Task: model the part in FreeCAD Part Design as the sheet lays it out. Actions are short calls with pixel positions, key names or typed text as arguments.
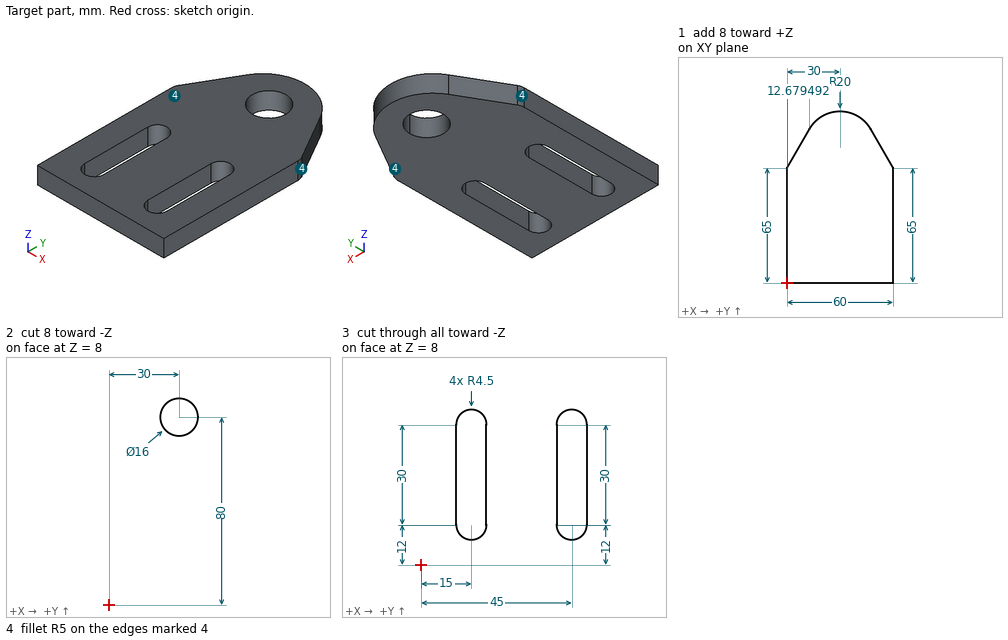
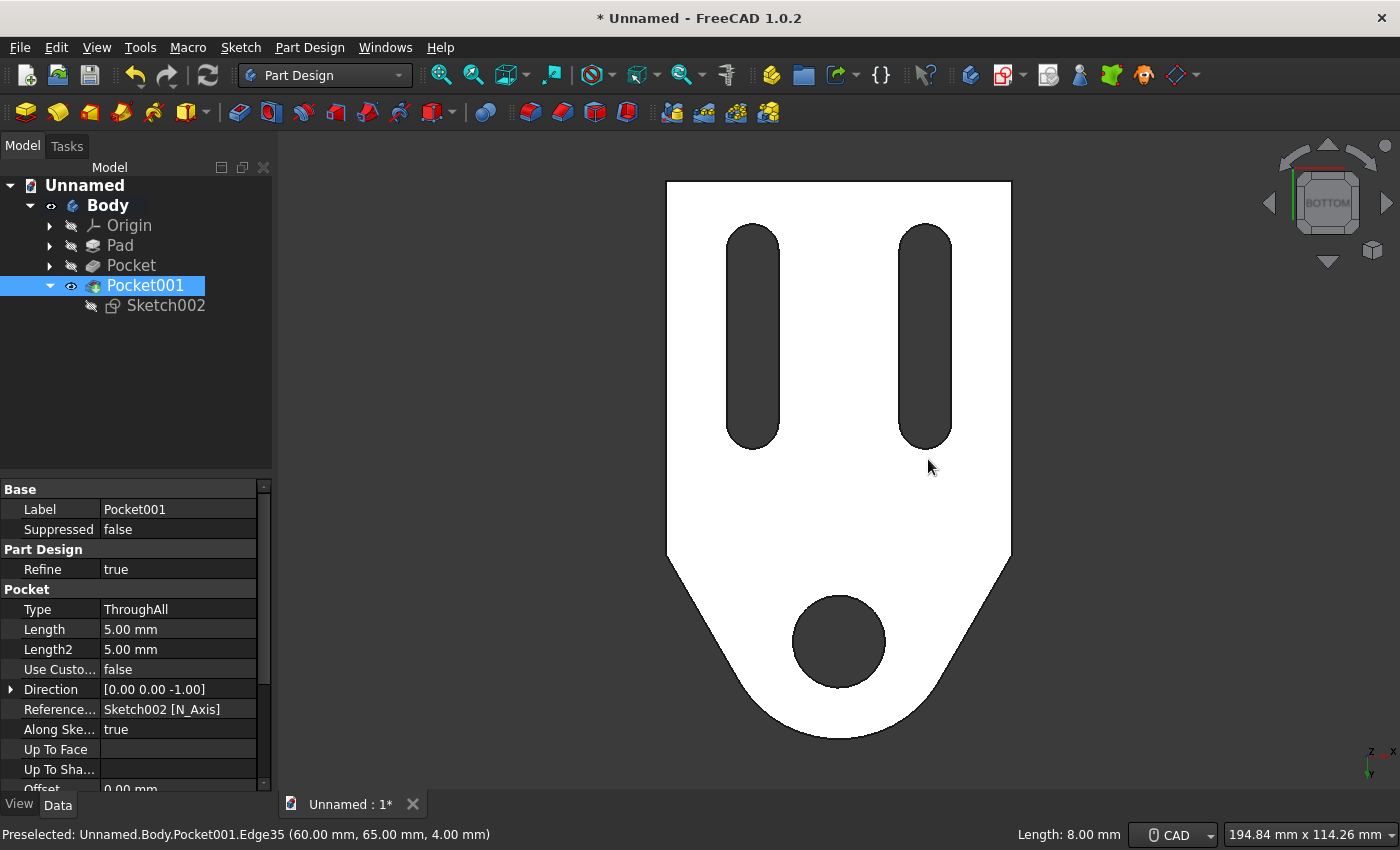
key(4)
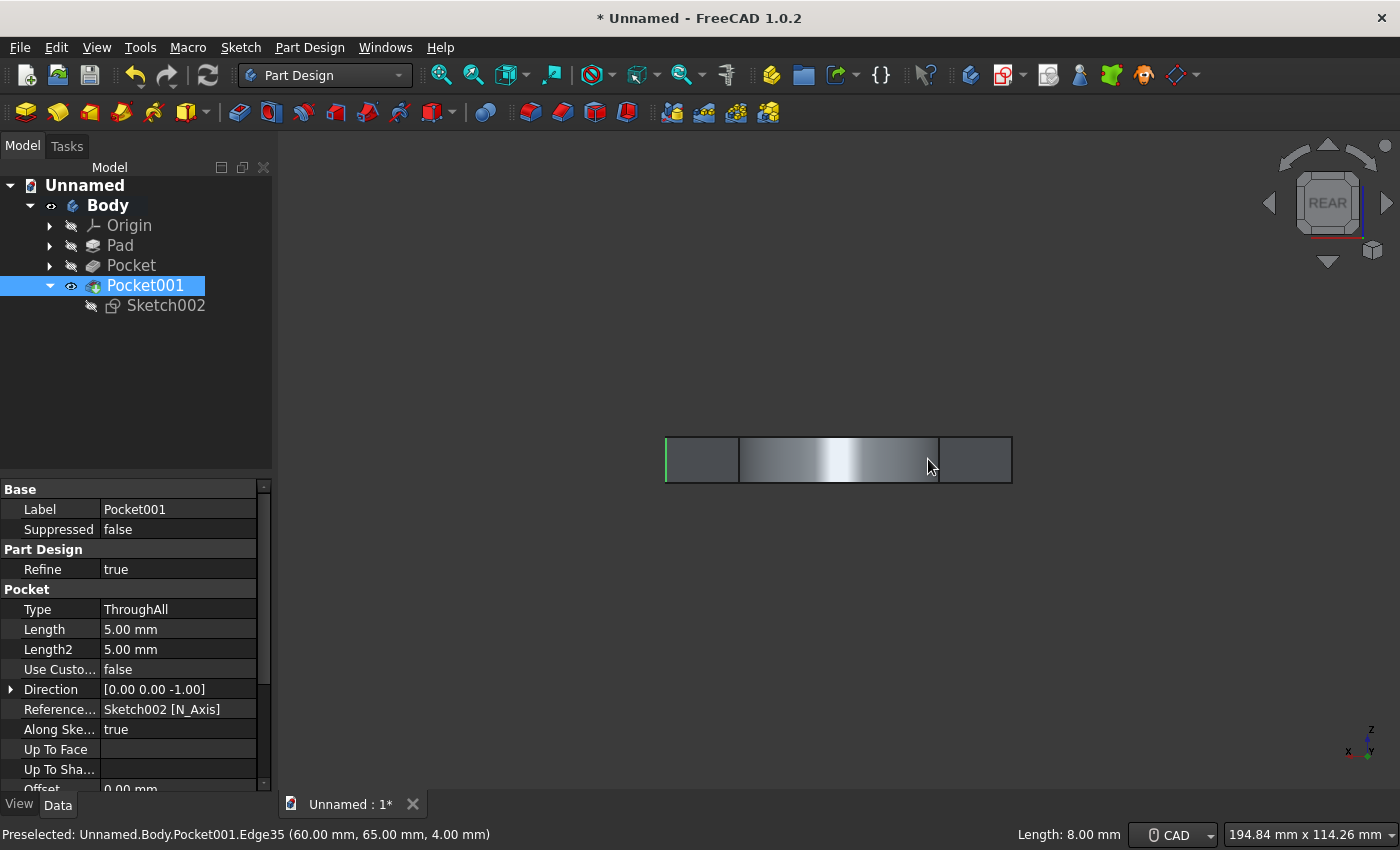
key(v)
key(f)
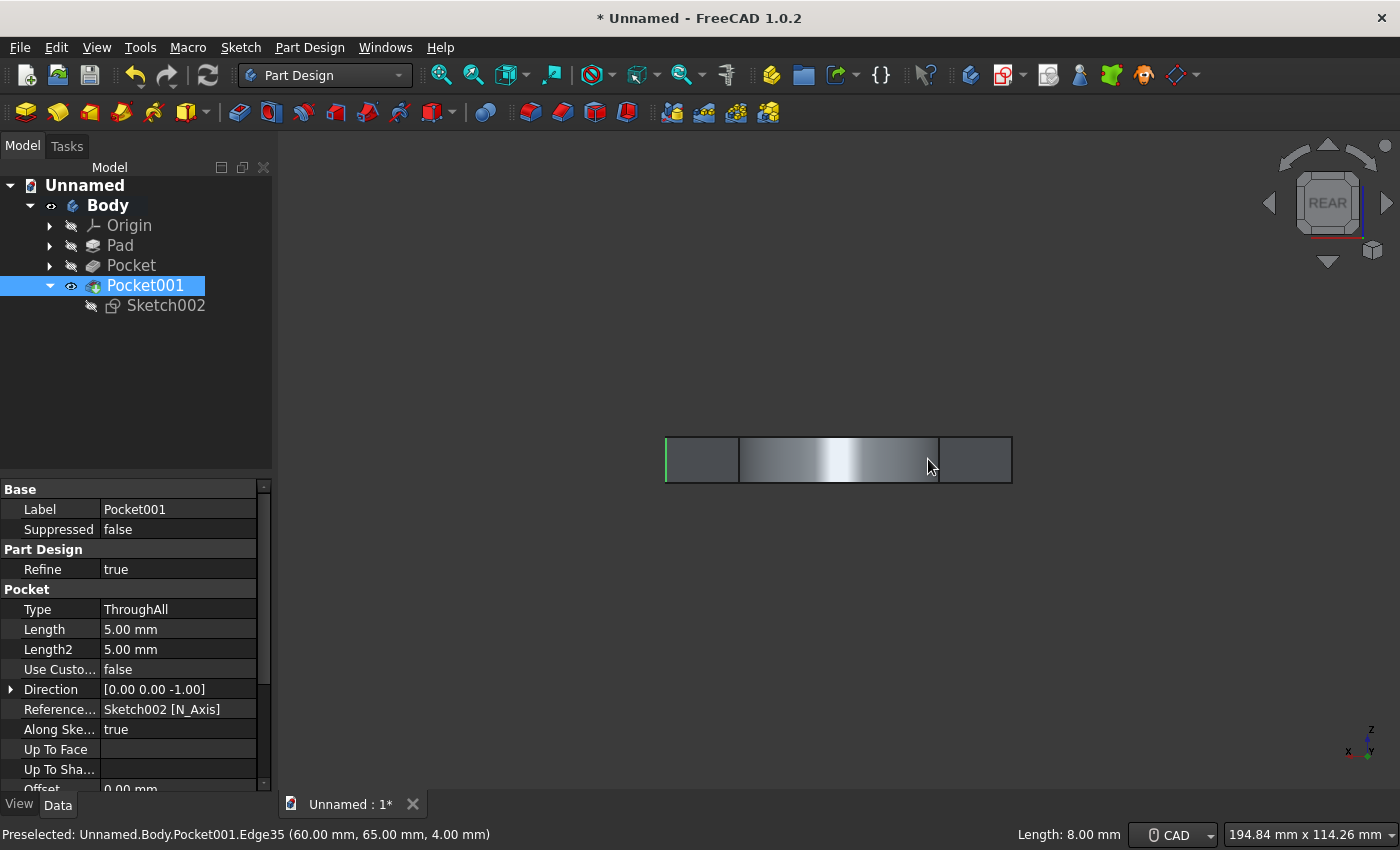
key(6)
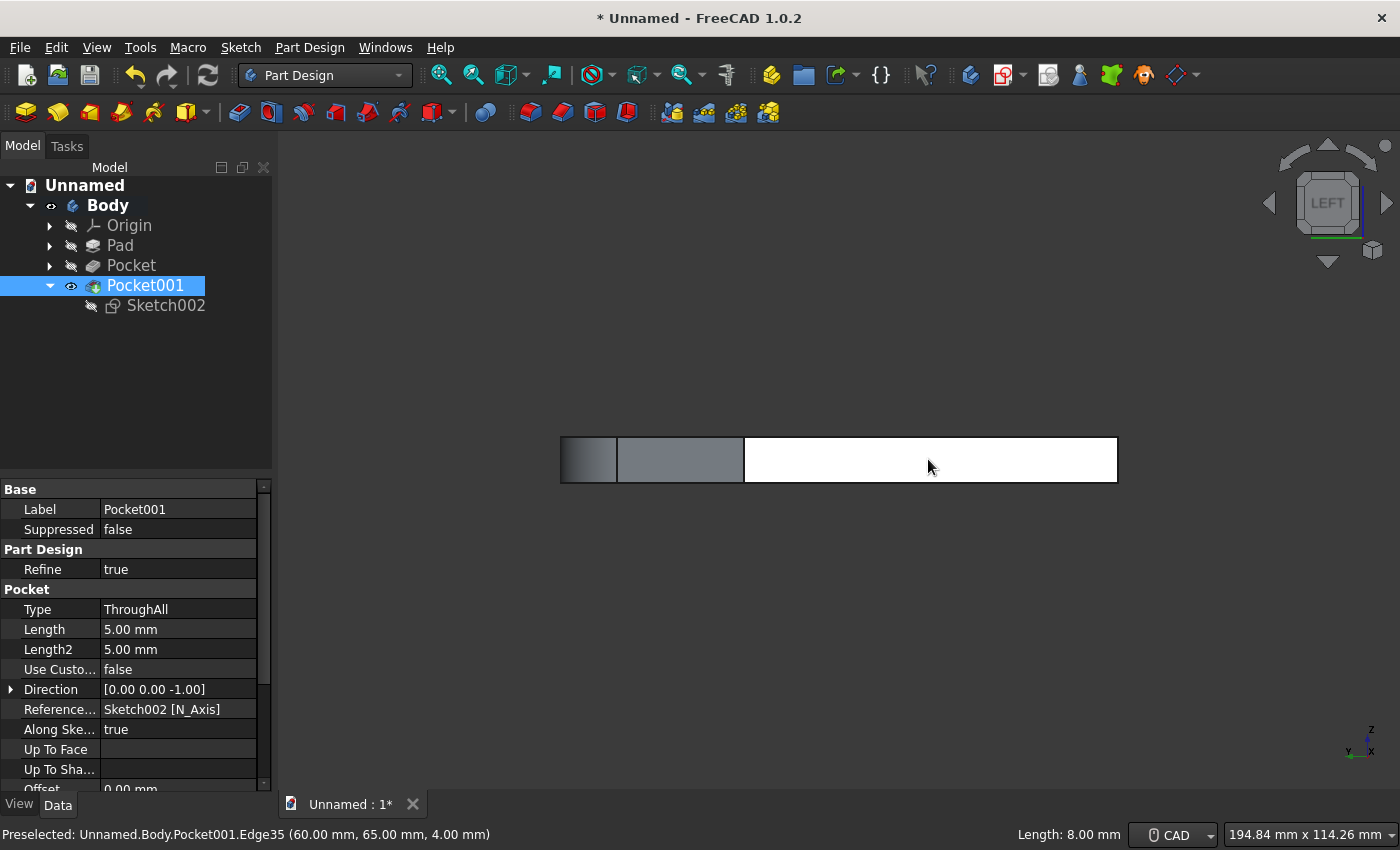
click(744, 459, ctrl)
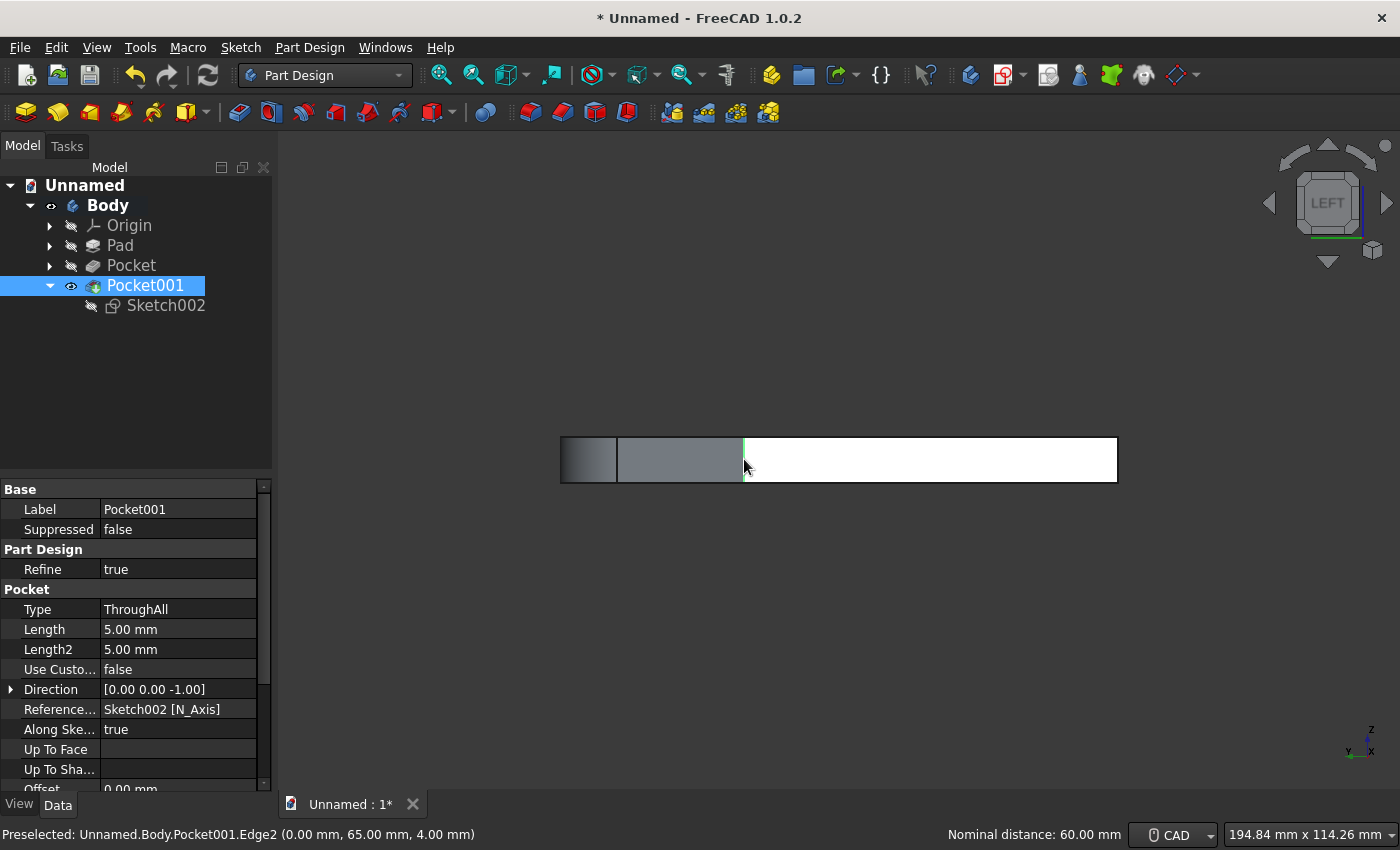
click(532, 112)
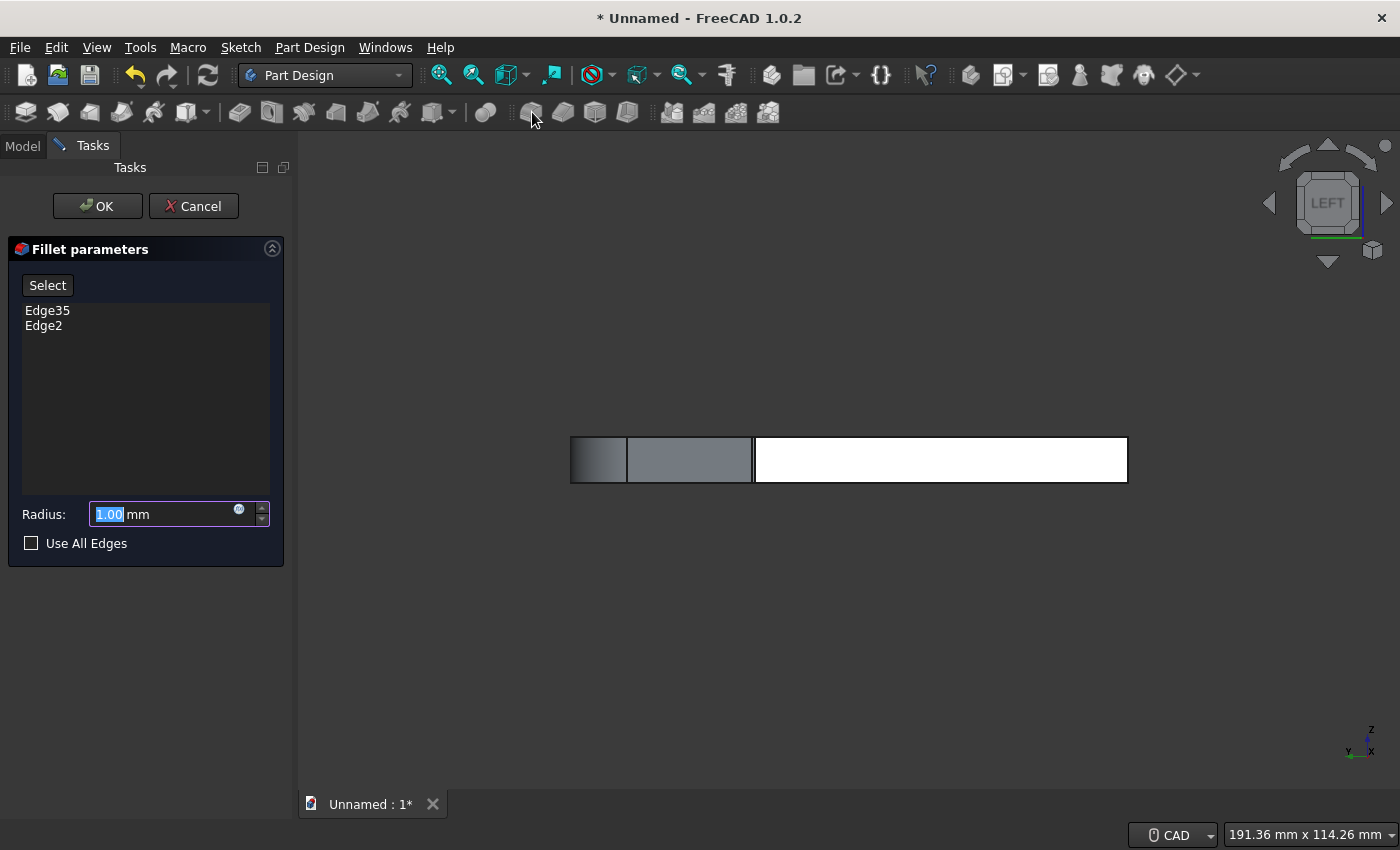
text(5)
key(Tab)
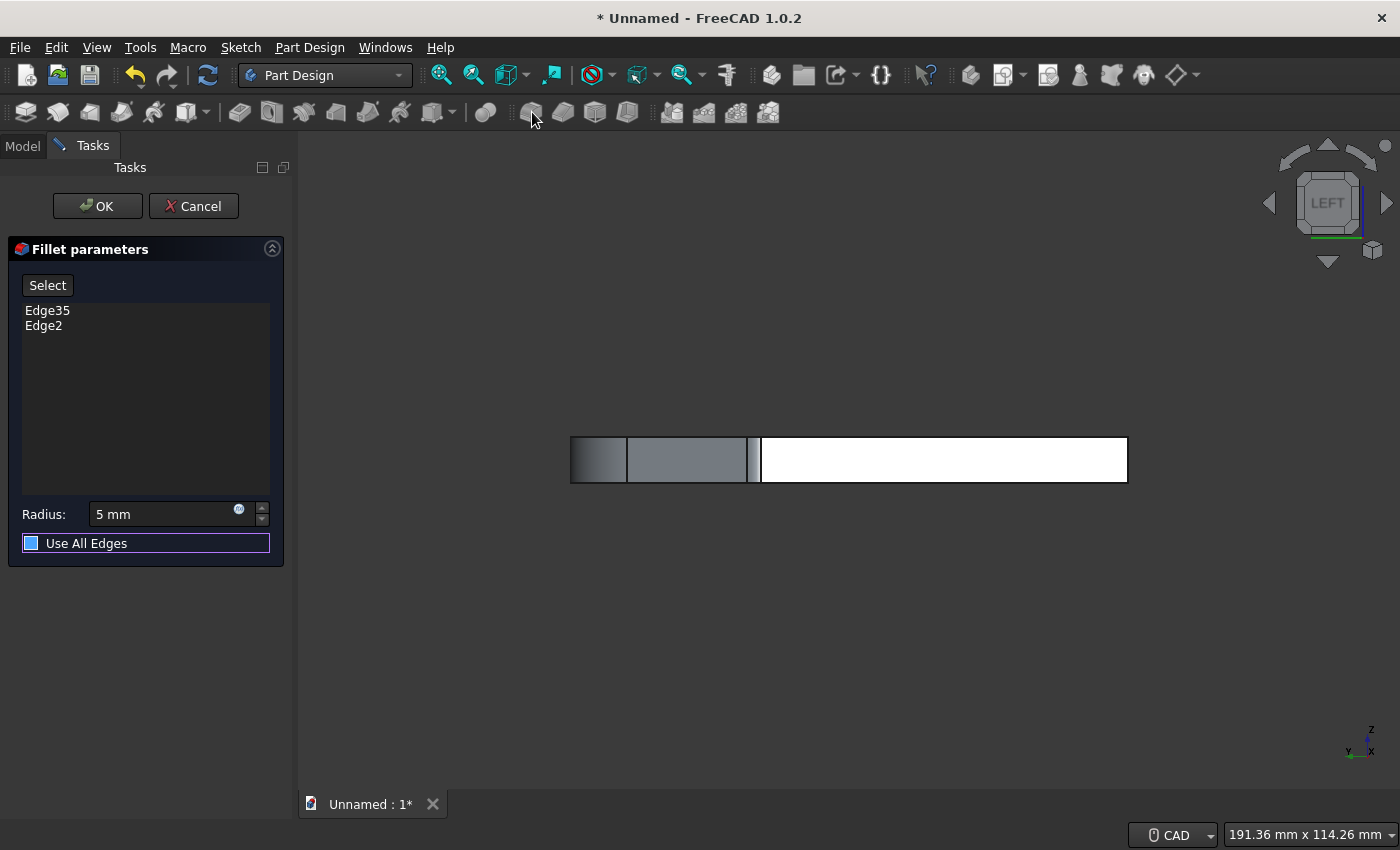
click(98, 206)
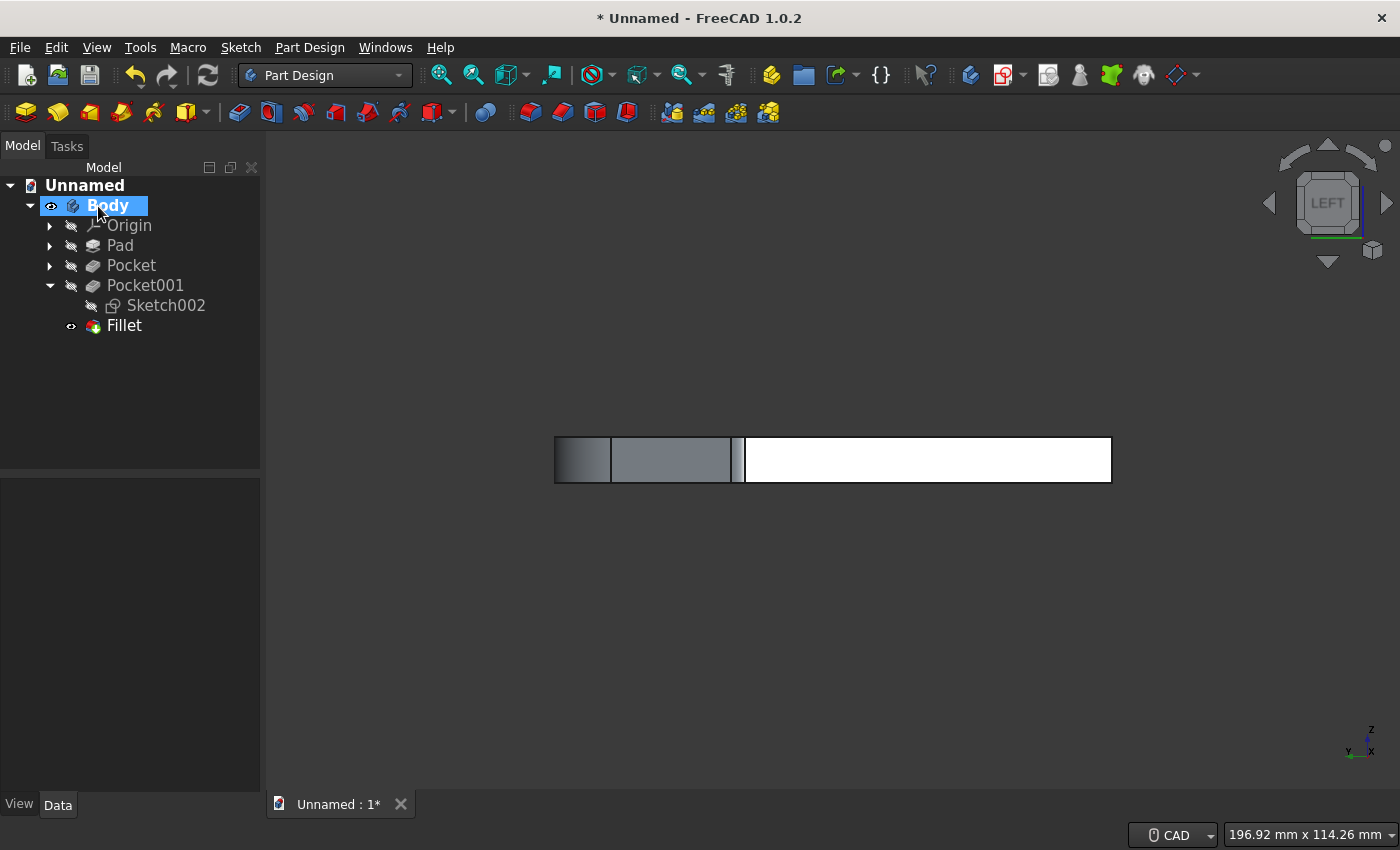
key(0)